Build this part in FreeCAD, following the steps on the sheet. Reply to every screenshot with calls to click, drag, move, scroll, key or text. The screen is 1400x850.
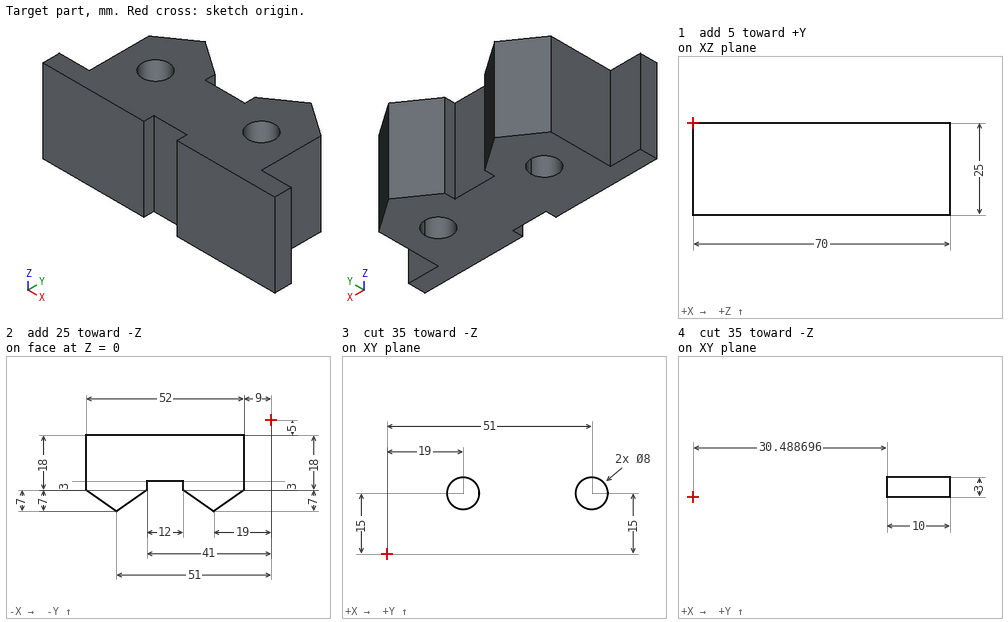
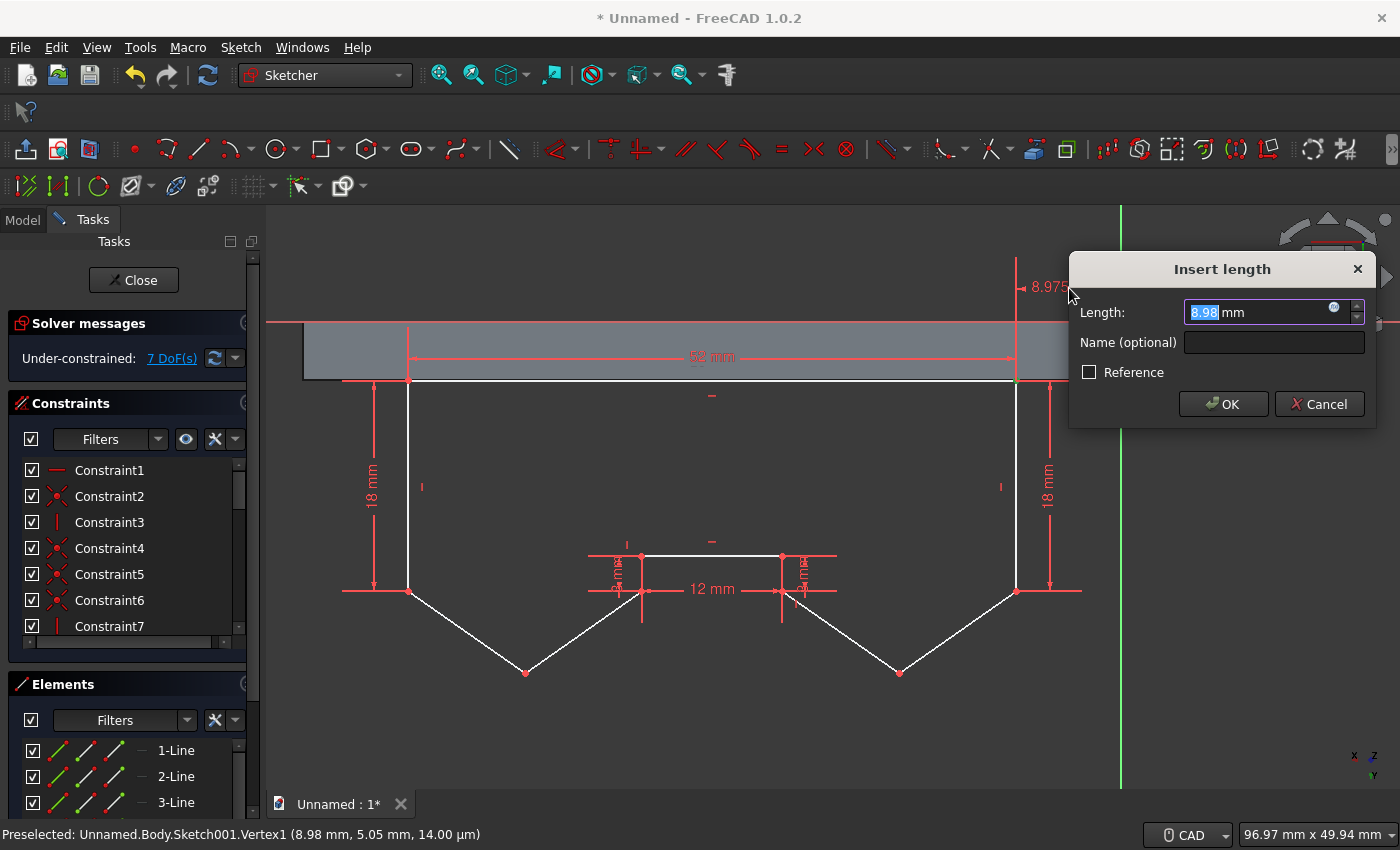
text(9)
key(Return)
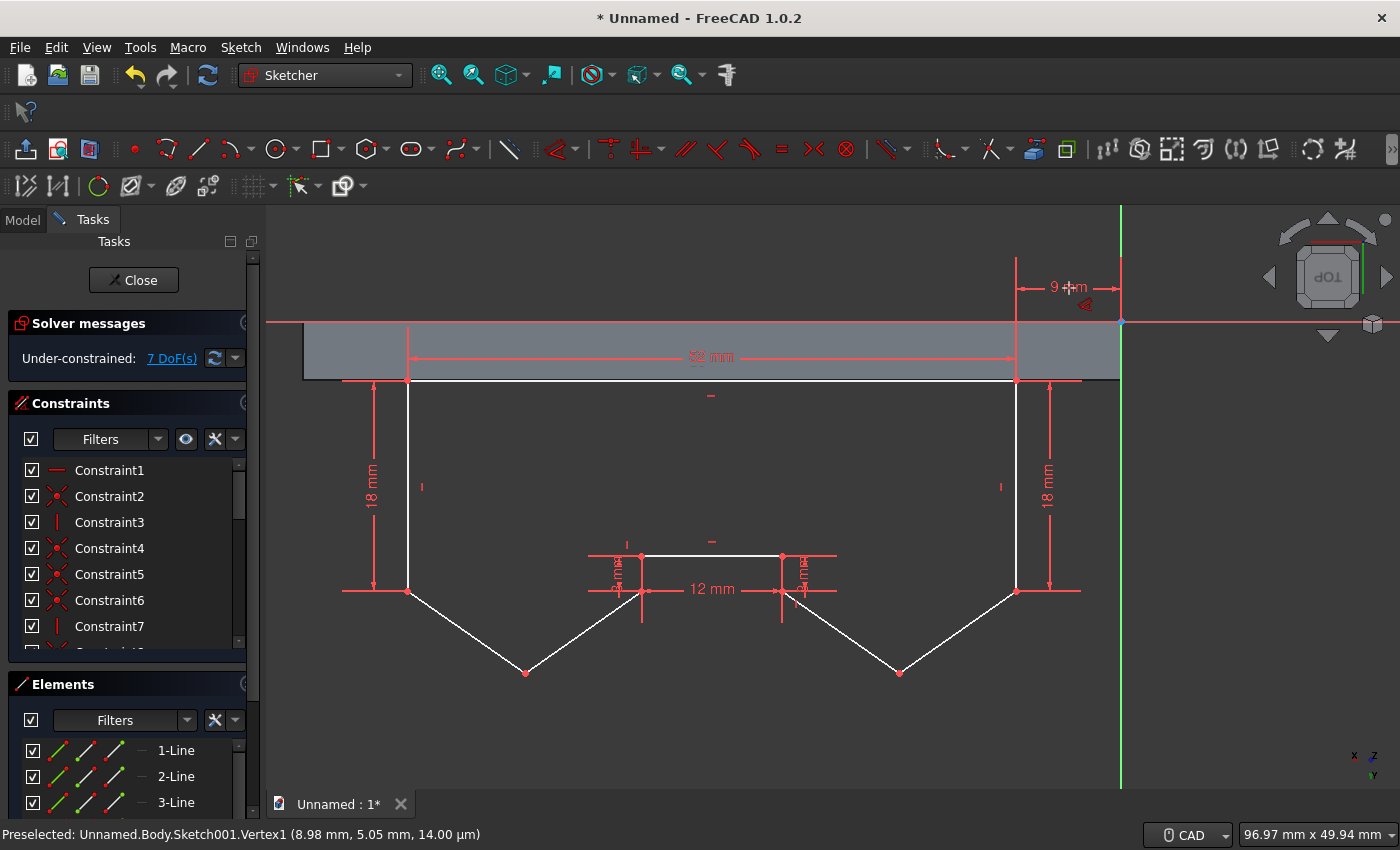
click(1016, 381)
click(1155, 351)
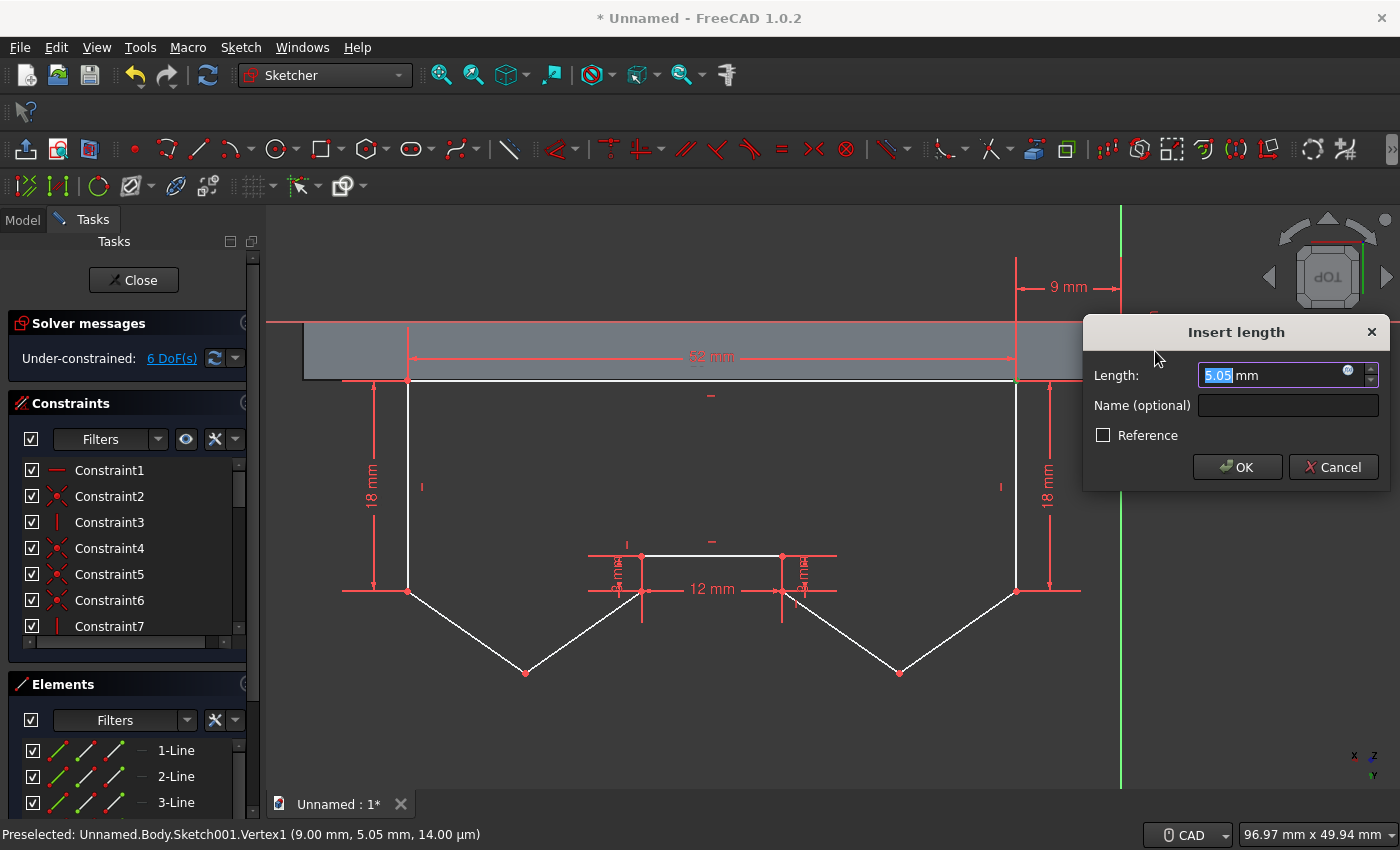
text(5)
key(Return)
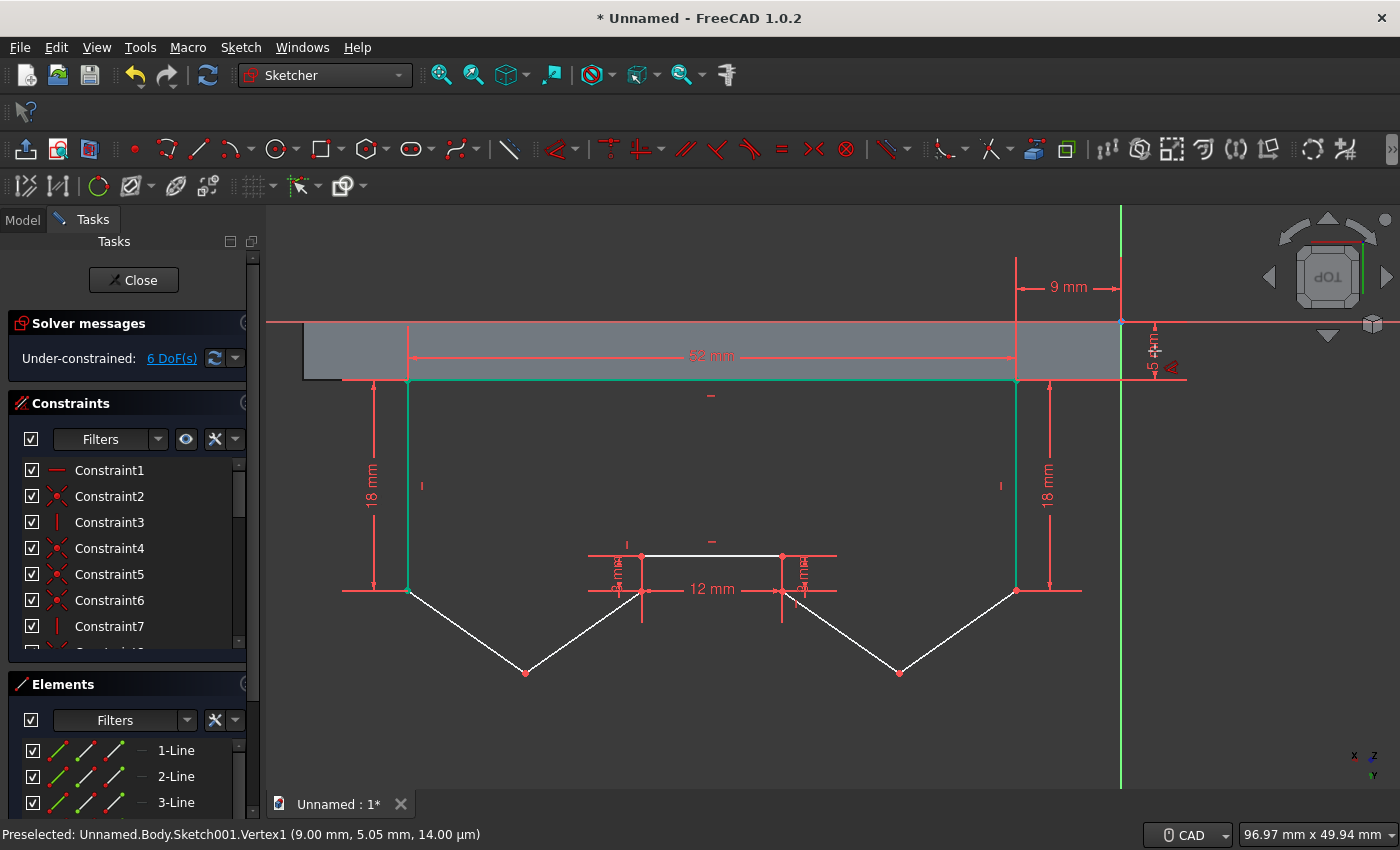
click(443, 616)
click(374, 632)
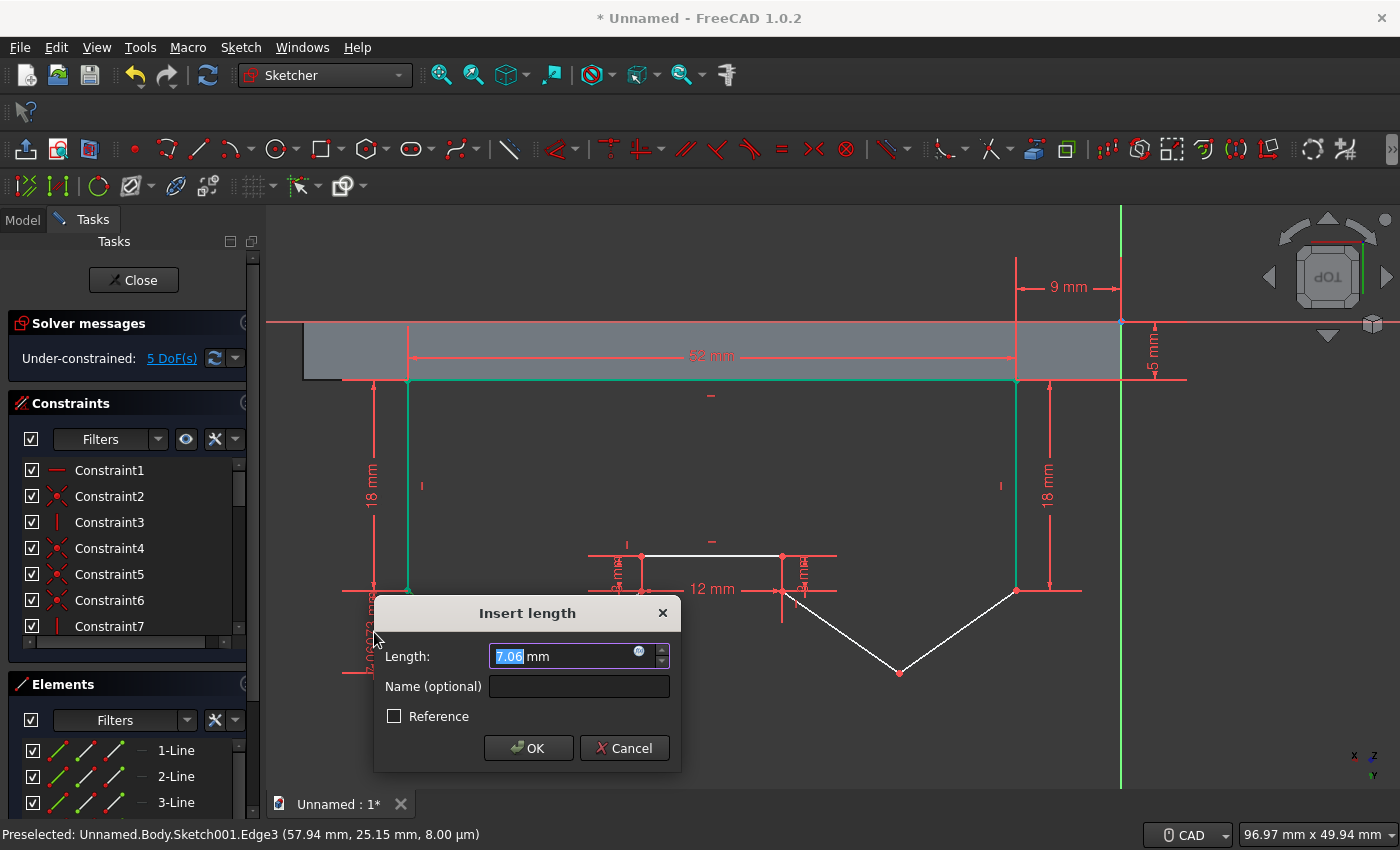
text(7)
key(Return)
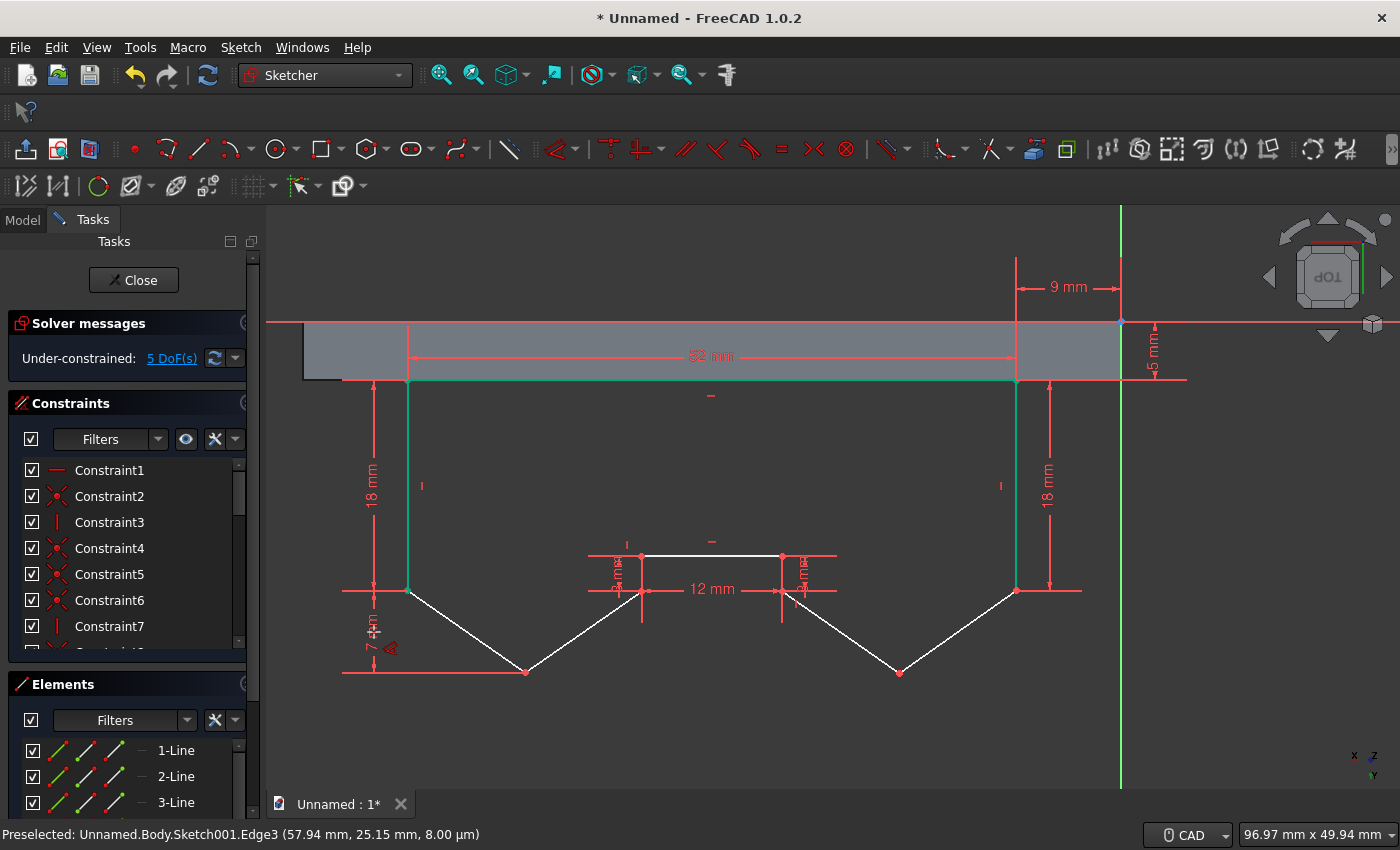
click(560, 648)
click(491, 632)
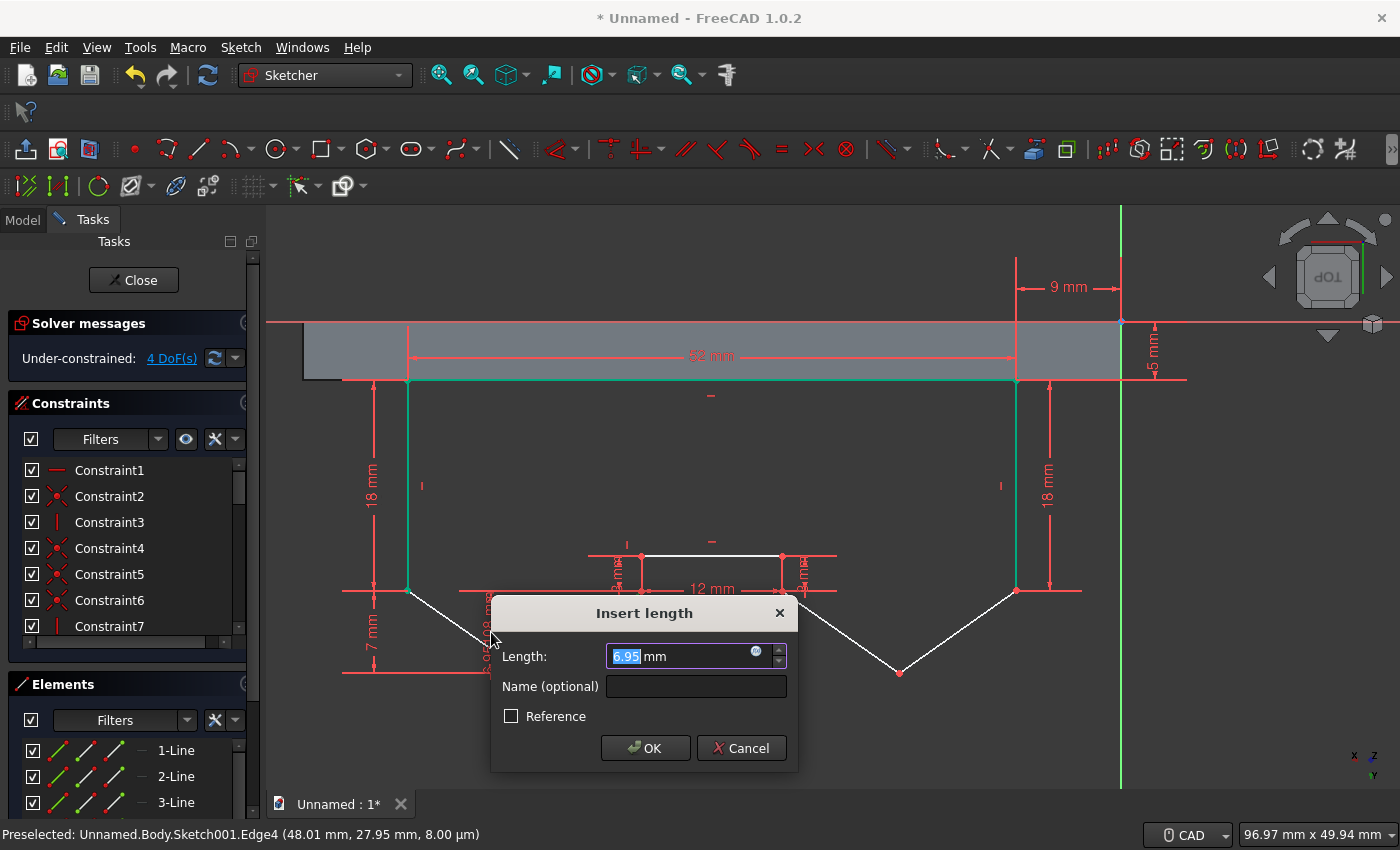
text(7)
key(Return)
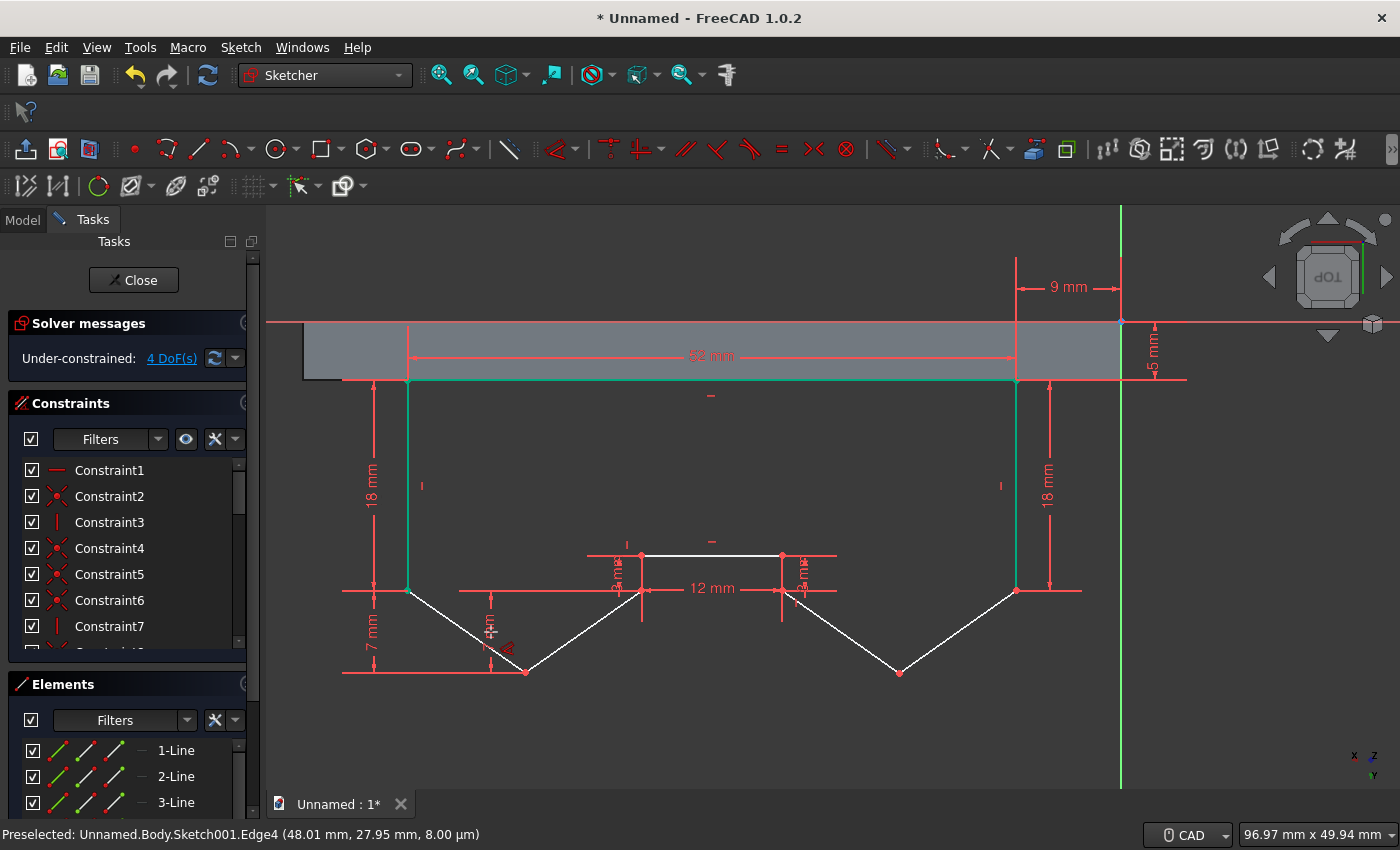
click(817, 616)
click(933, 632)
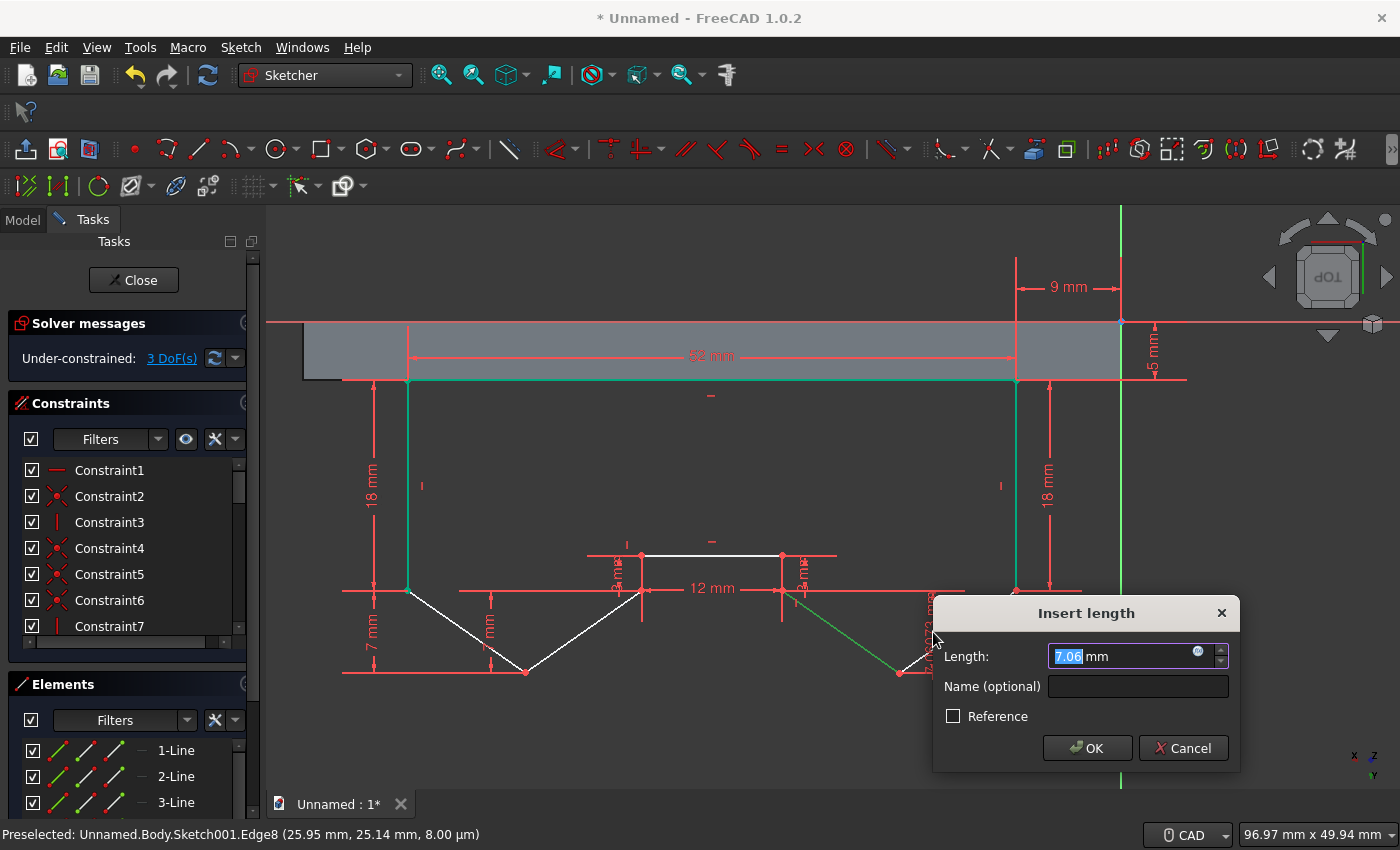
text(7)
key(Return)